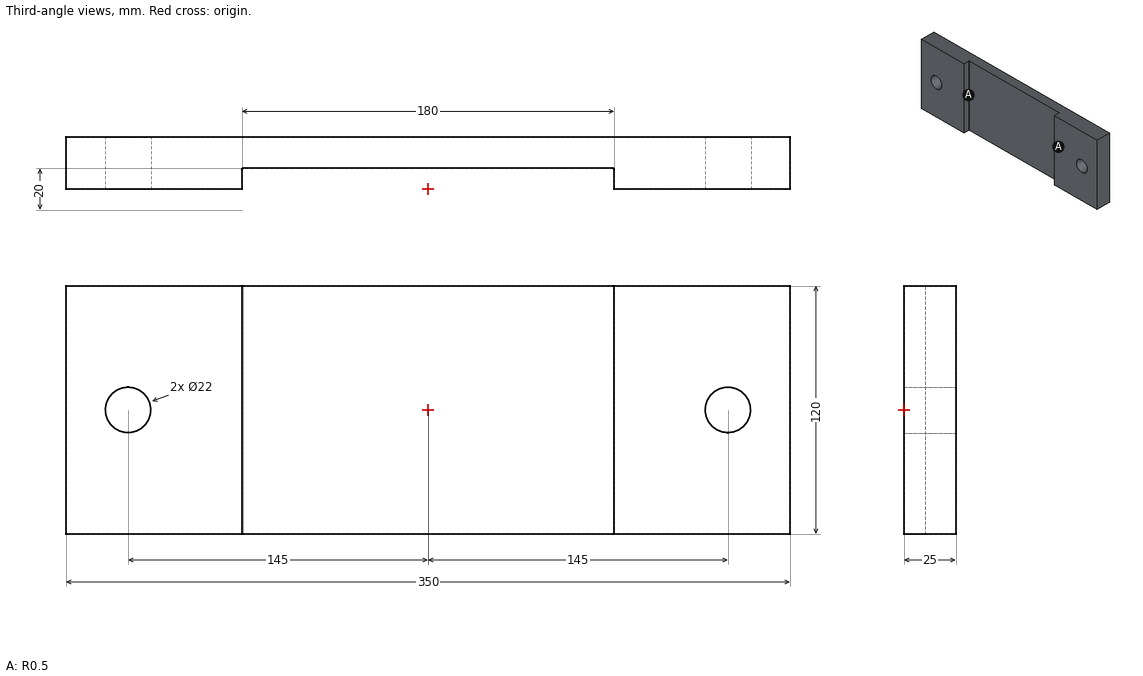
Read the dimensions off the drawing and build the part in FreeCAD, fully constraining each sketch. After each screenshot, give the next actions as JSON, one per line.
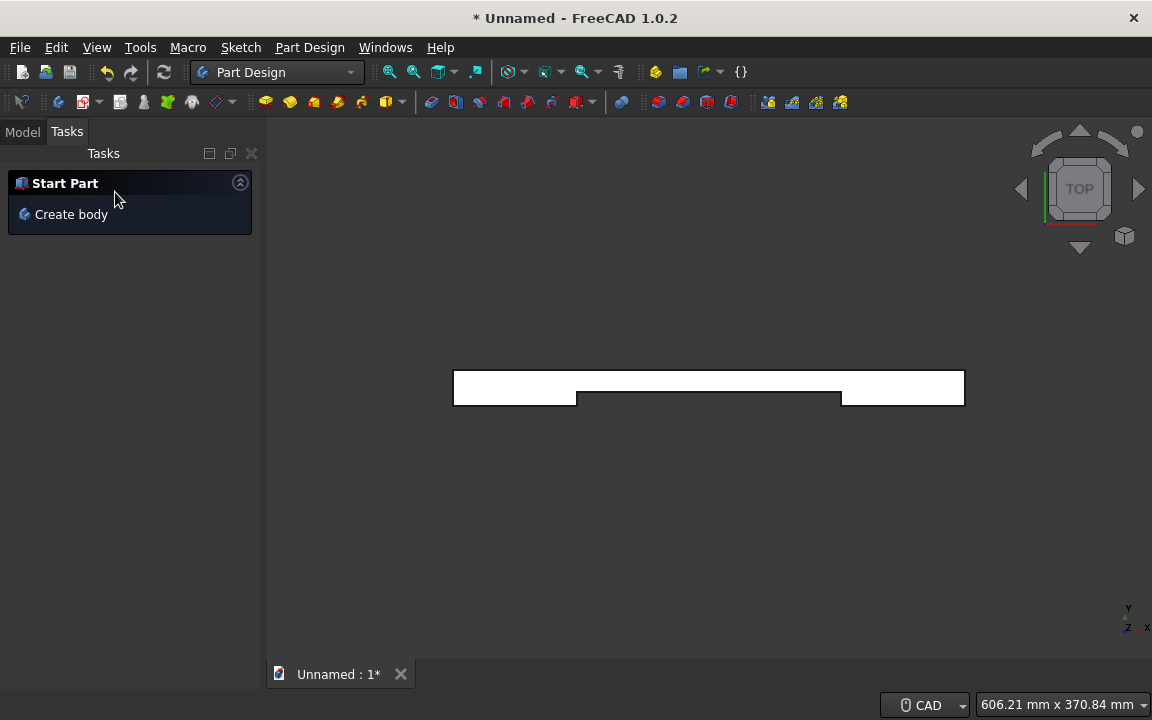
{"action": "key", "text": "1"}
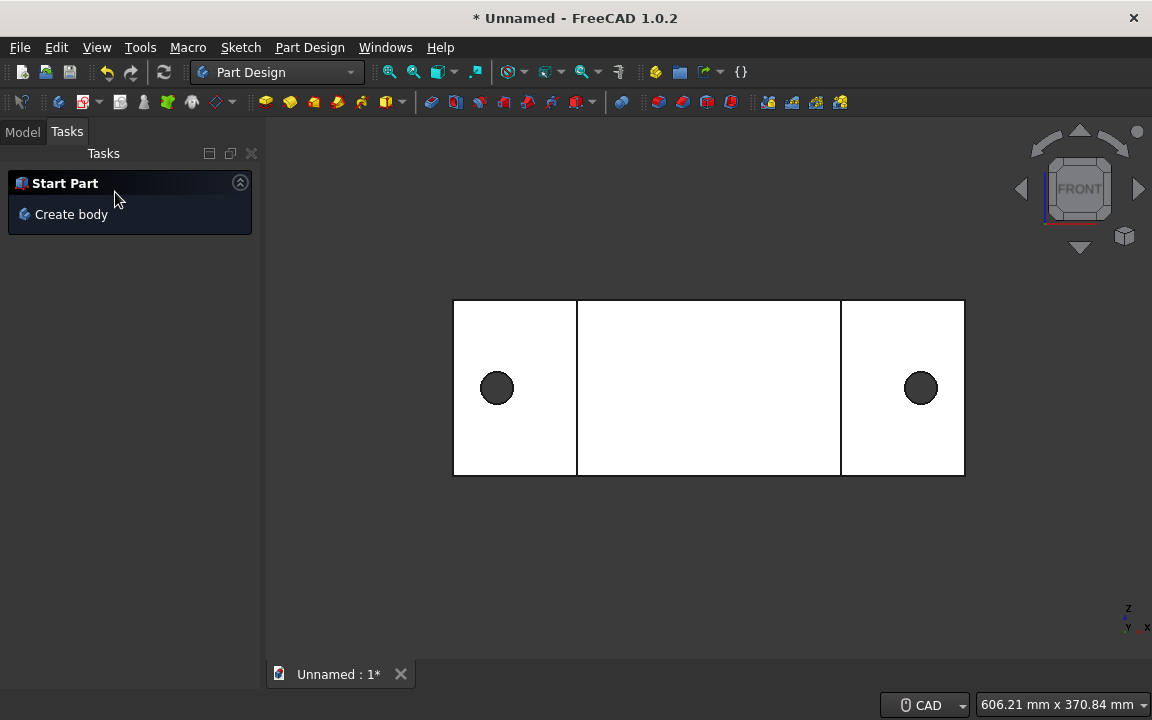
{"action": "key", "text": "3"}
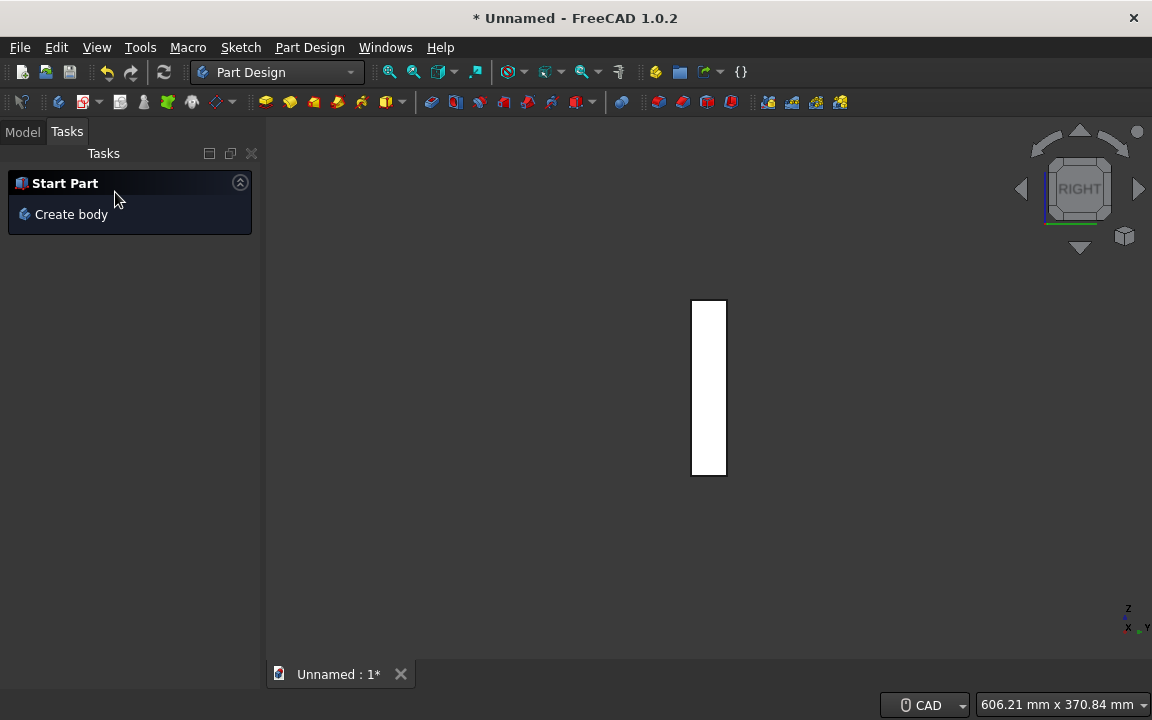
{"action": "left_click", "coordinate": [390, 72]}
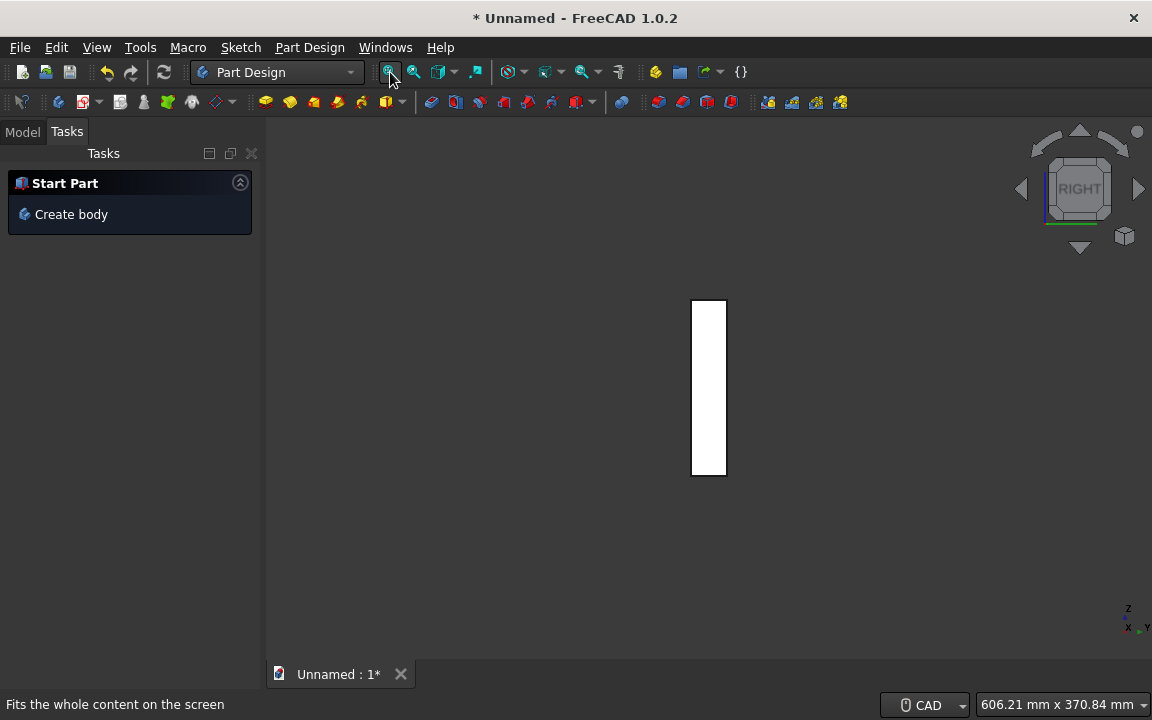
{"action": "key", "text": "5"}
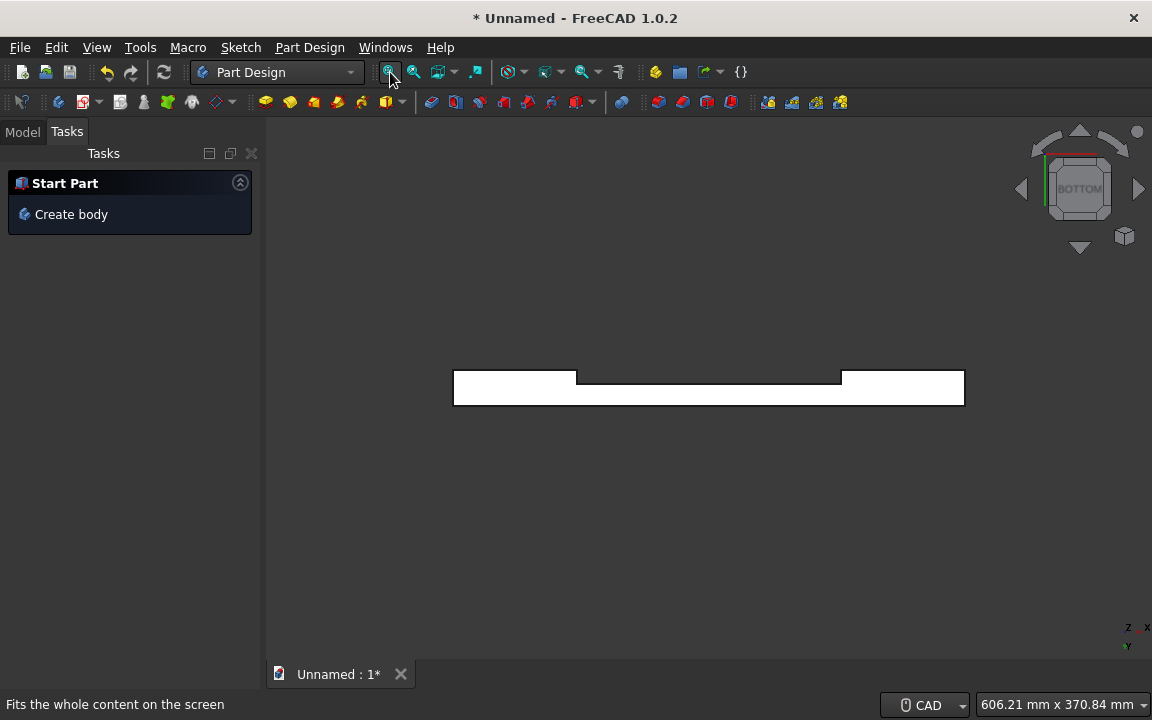
{"action": "key", "text": "4"}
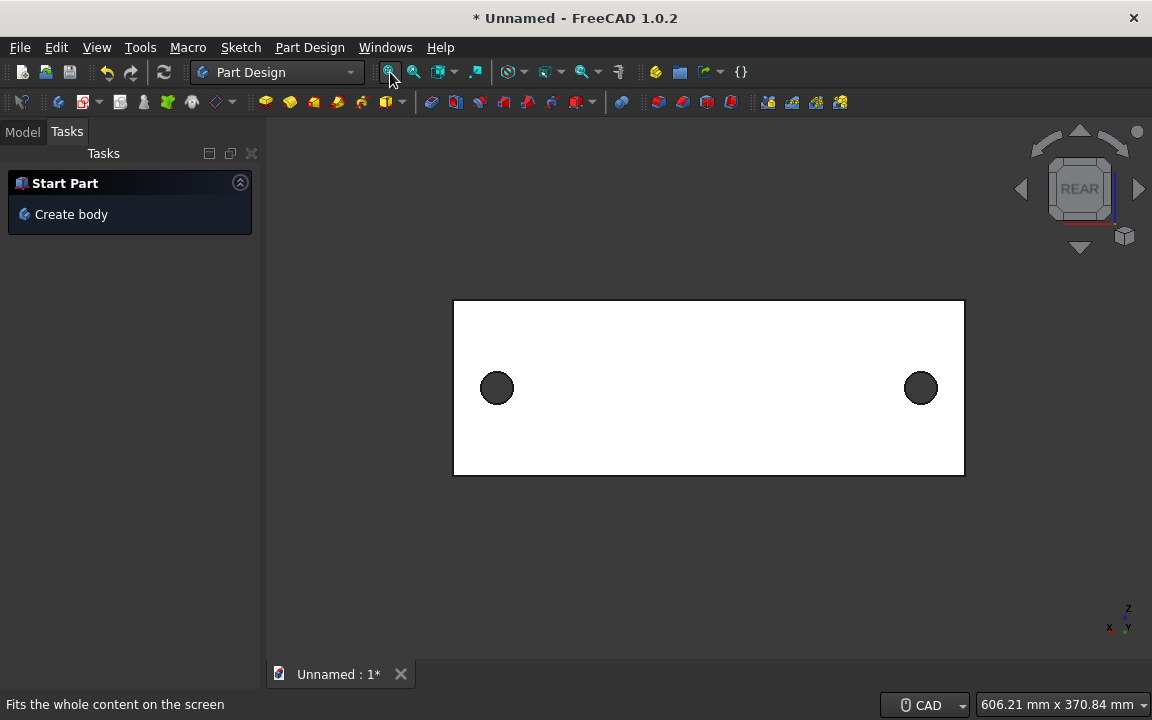
{"action": "key", "text": "6"}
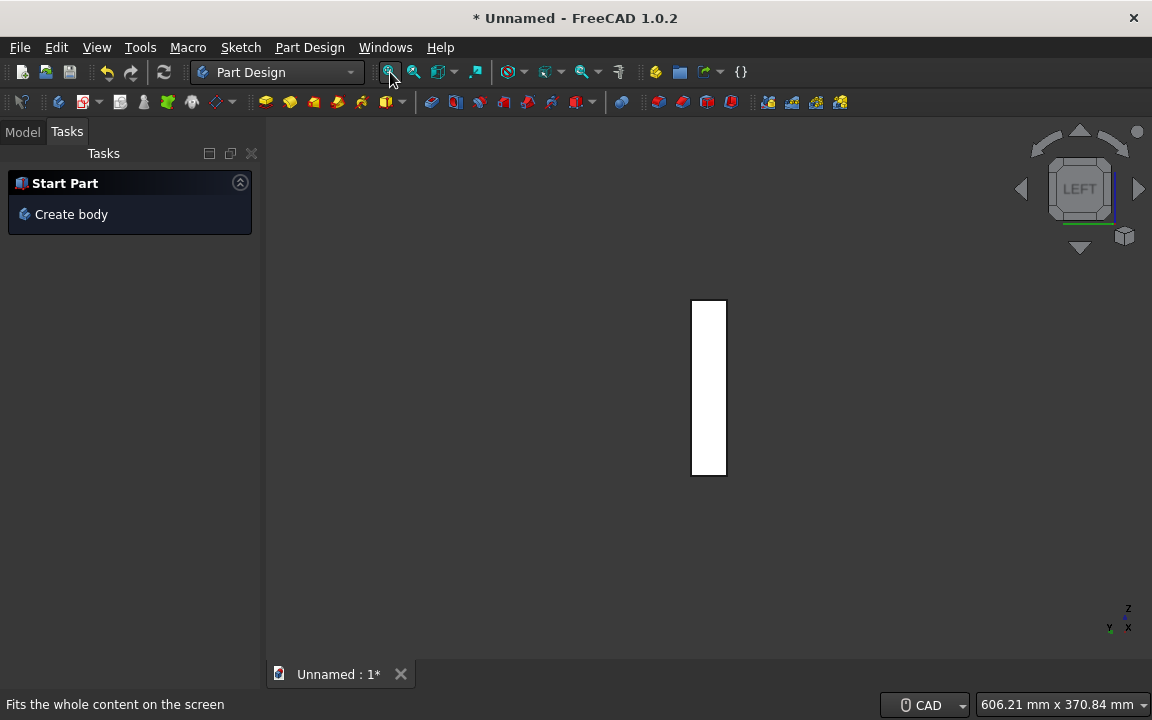
{"action": "left_click", "coordinate": [390, 72]}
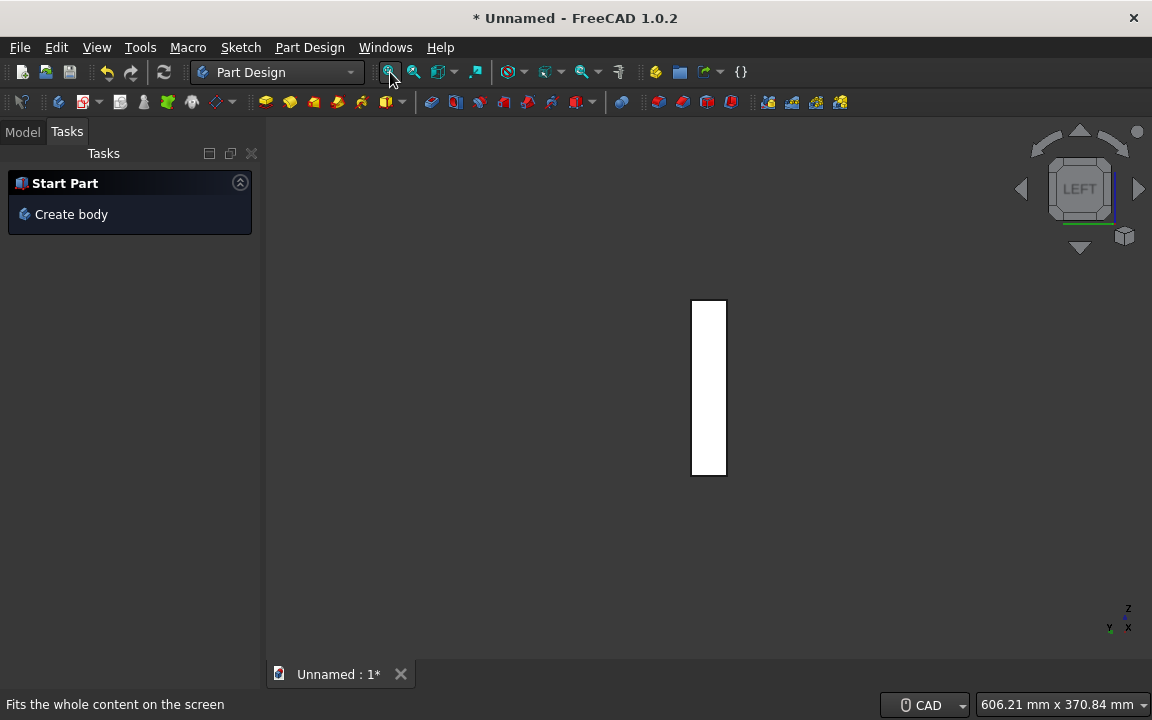
{"action": "key", "text": "v 3"}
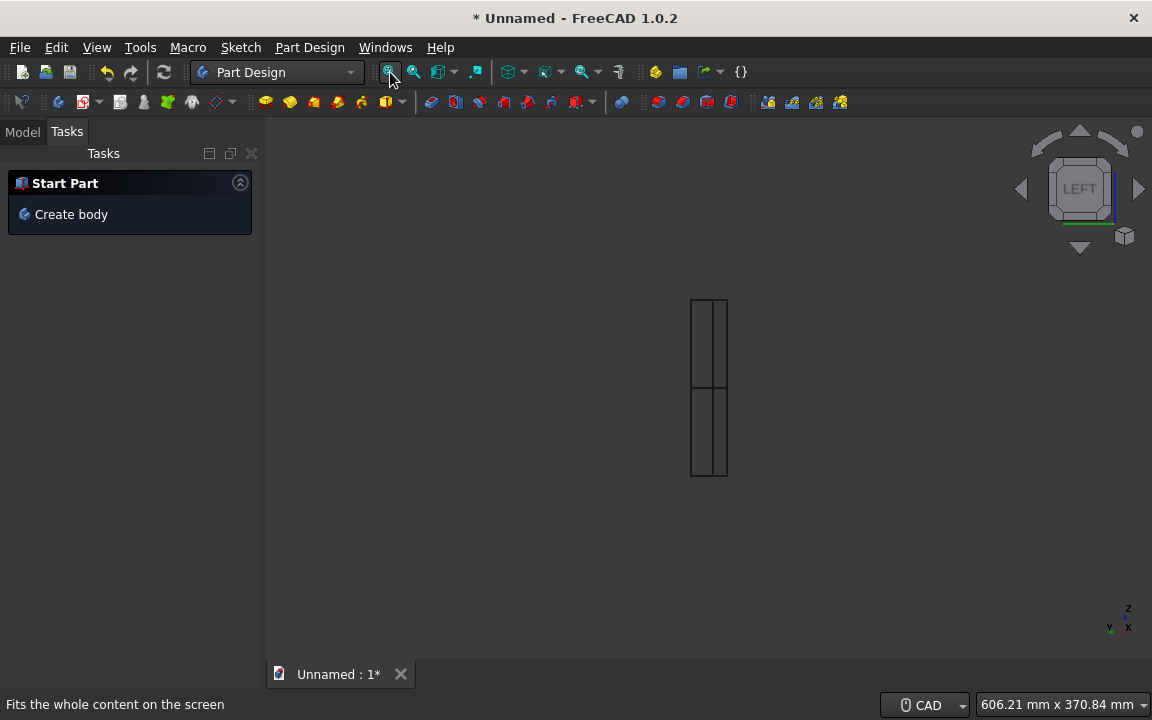
{"action": "key", "text": "0"}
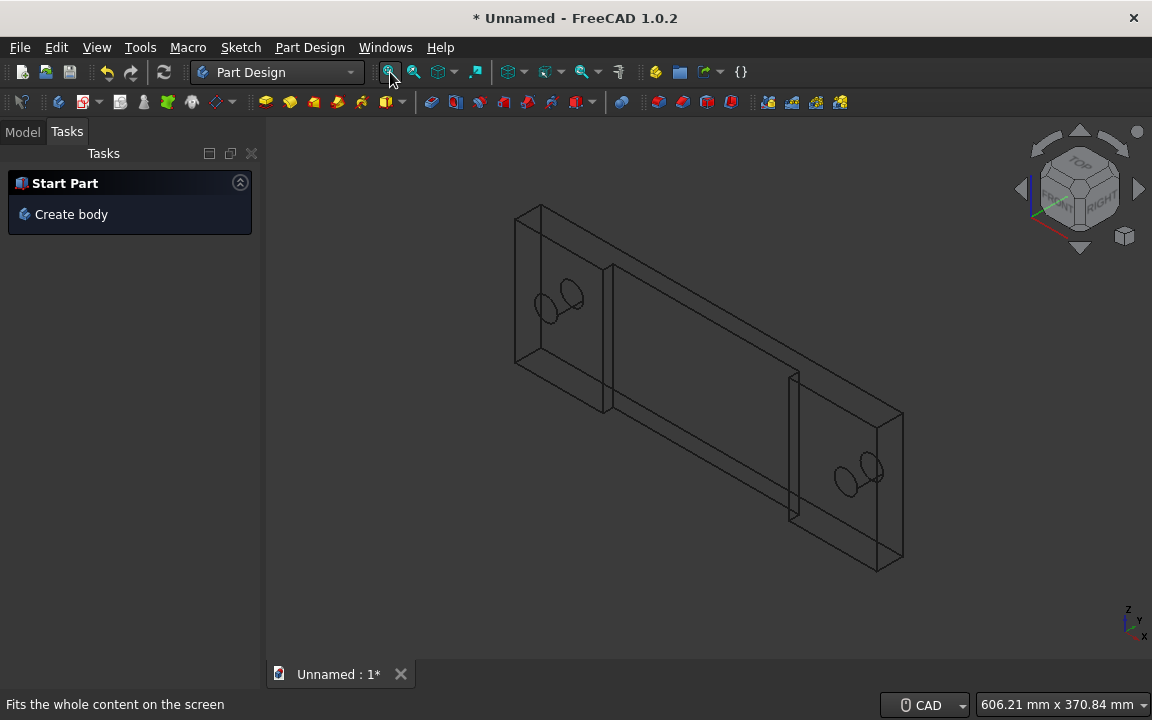
{"action": "left_click", "coordinate": [799, 442]}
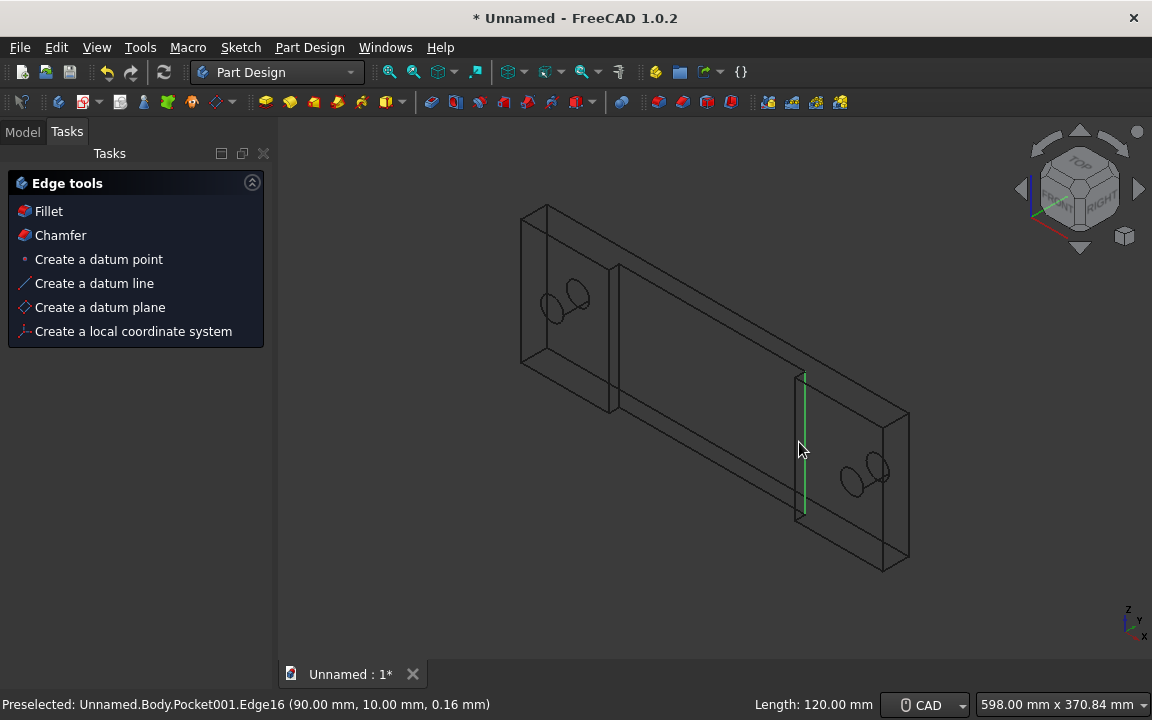
{"action": "left_click", "coordinate": [619, 335], "text": "ctrl"}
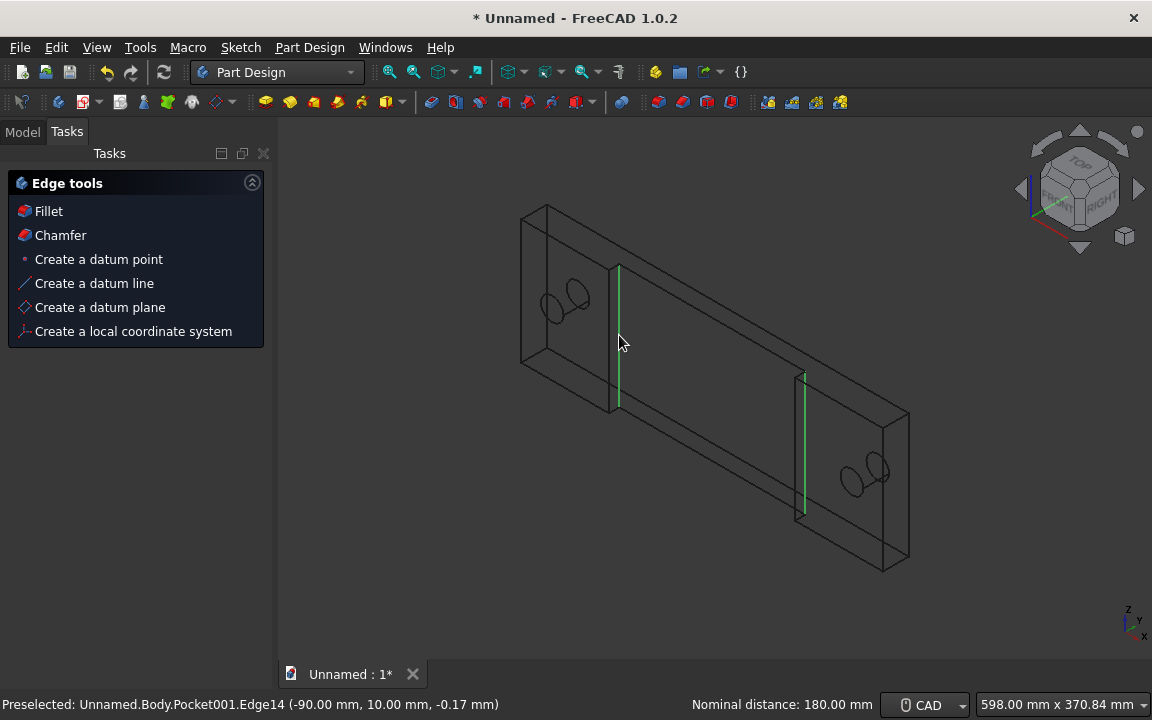
{"action": "key", "text": "v 1"}